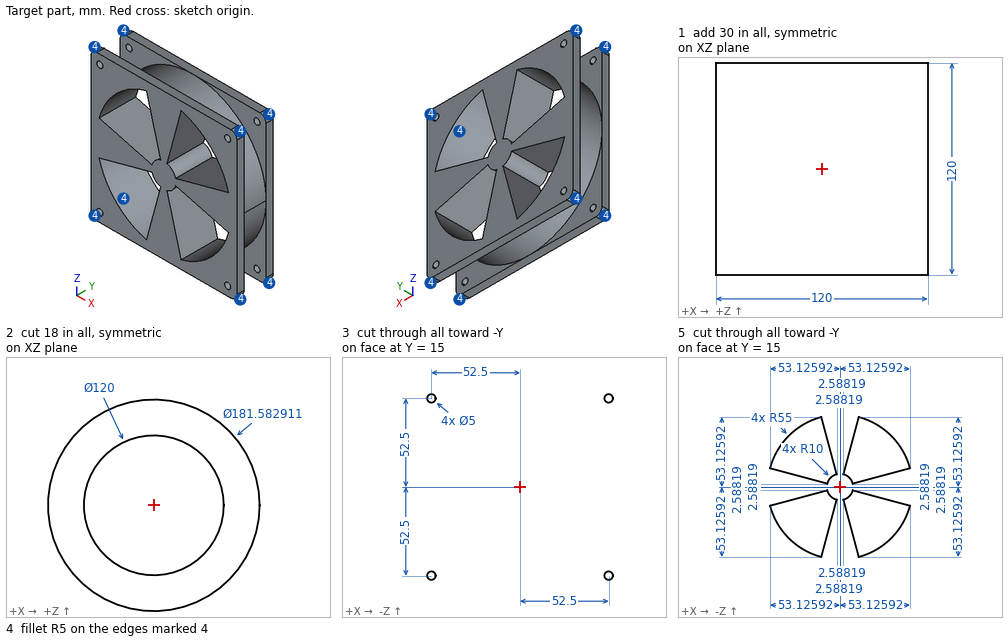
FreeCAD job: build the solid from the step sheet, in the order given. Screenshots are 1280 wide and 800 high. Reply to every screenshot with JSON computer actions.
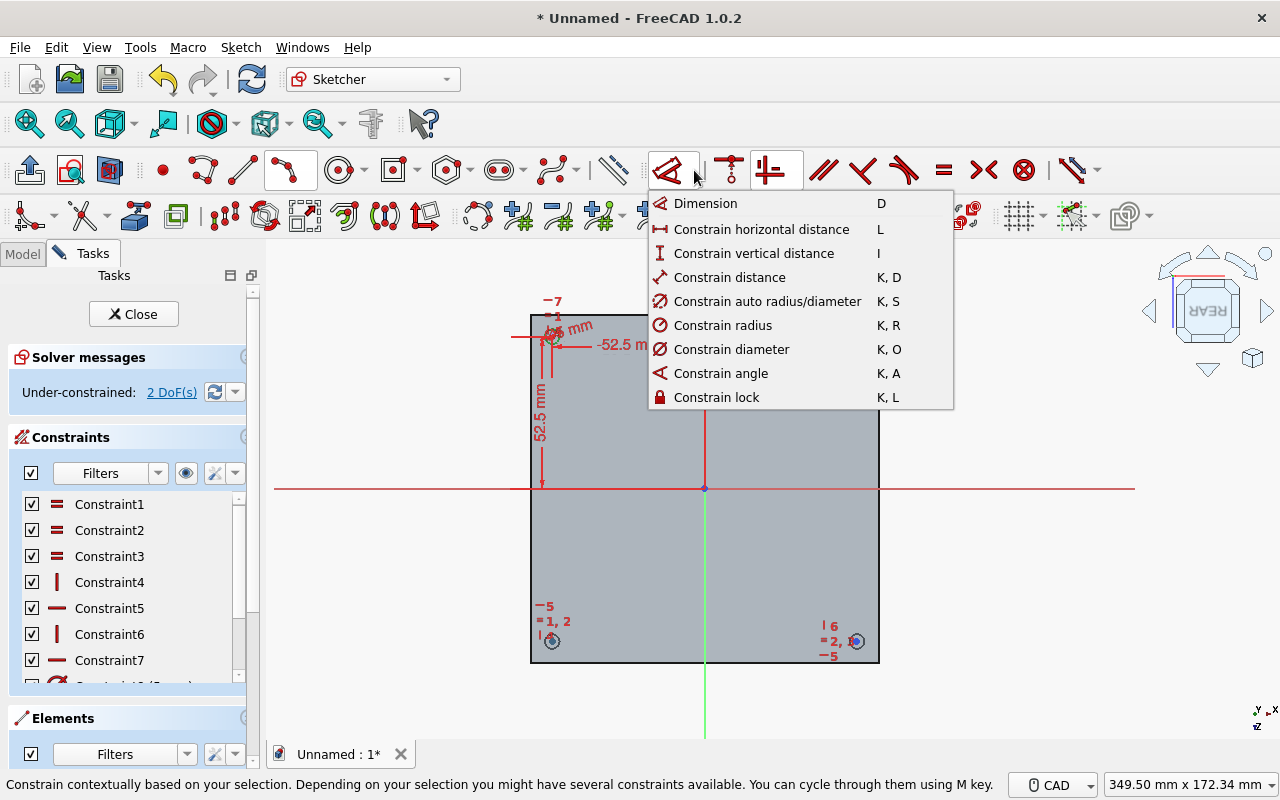
{"action": "left_click", "coordinate": [801, 253]}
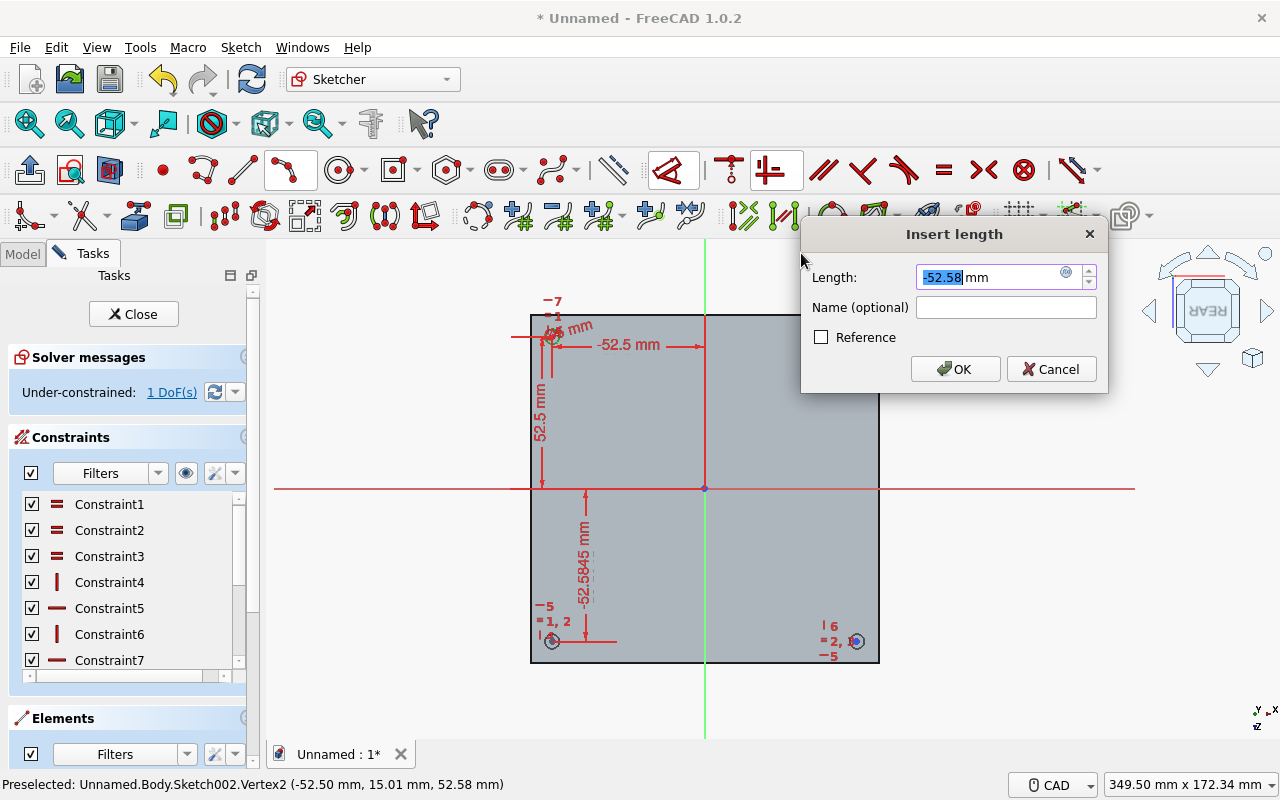
{"action": "type", "text": "-52.5"}
{"action": "key", "text": "Return"}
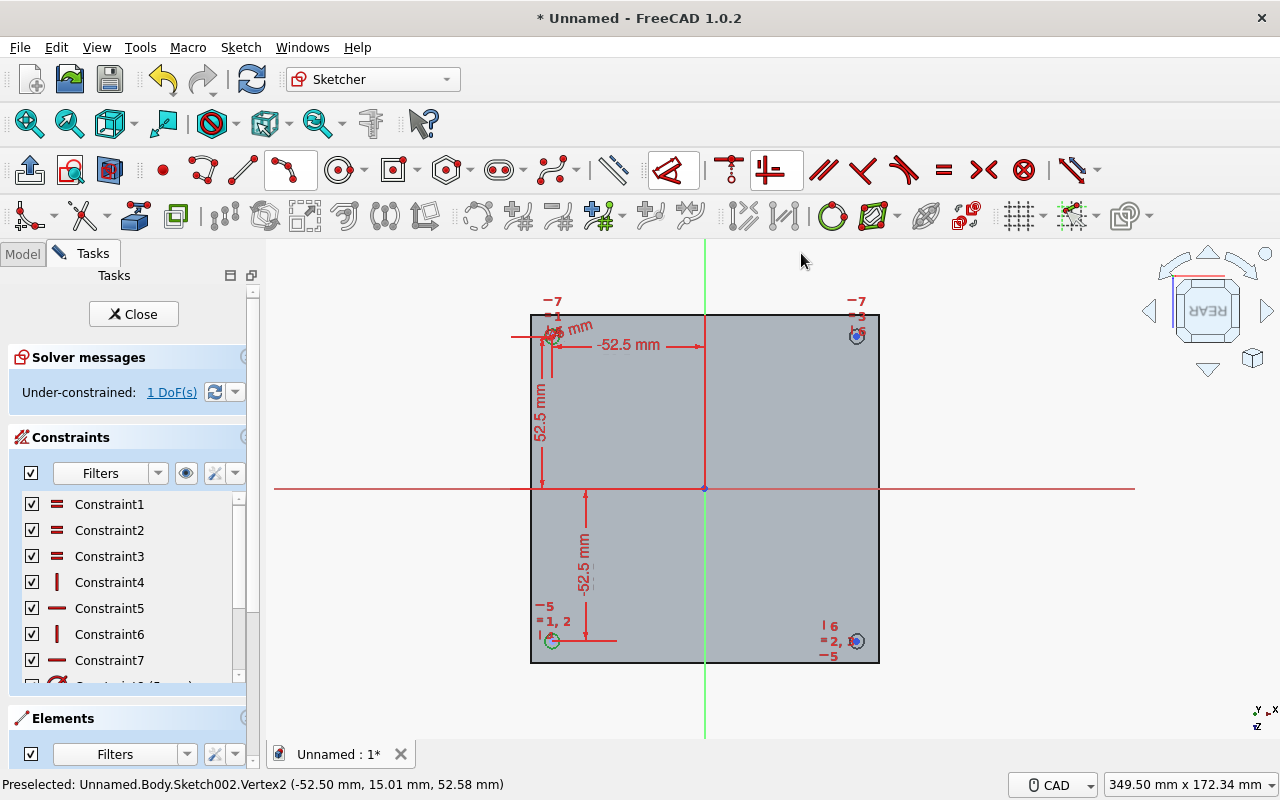
{"action": "left_click", "coordinate": [857, 641]}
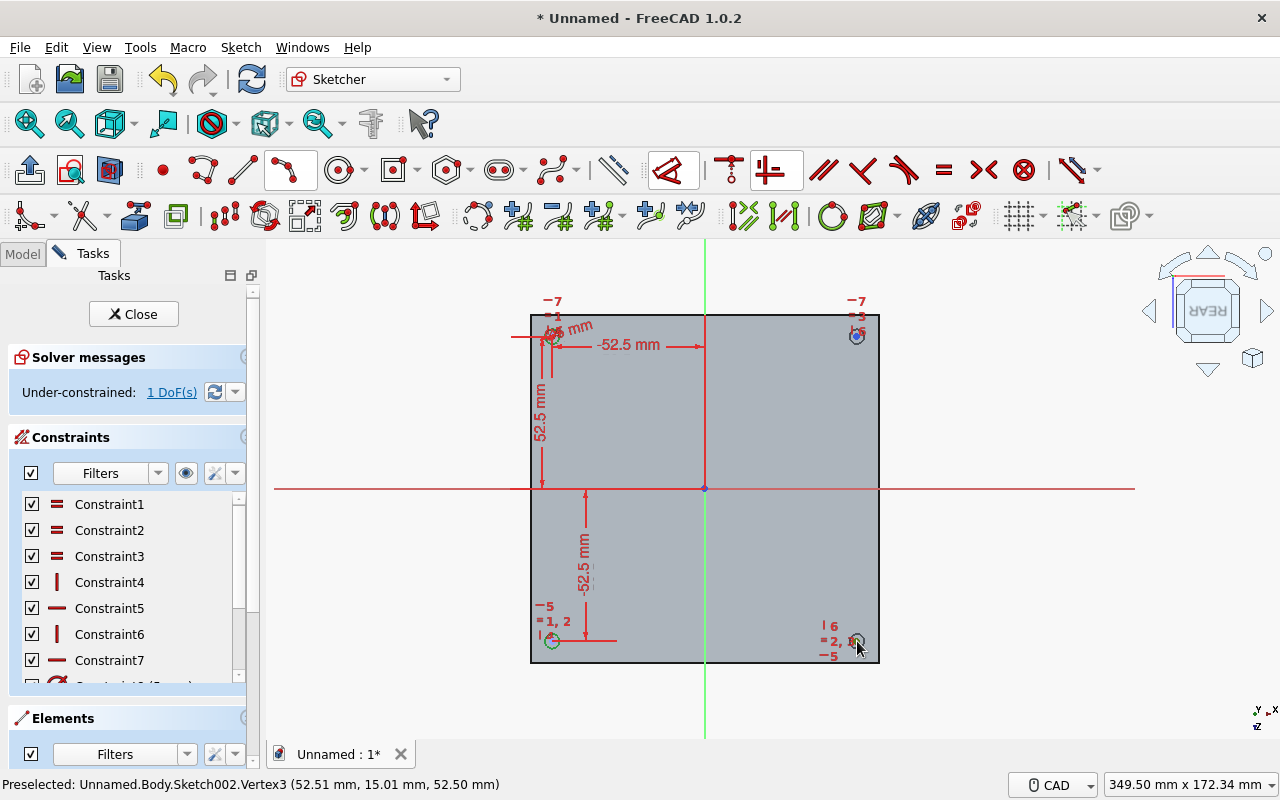
{"action": "key", "text": "l"}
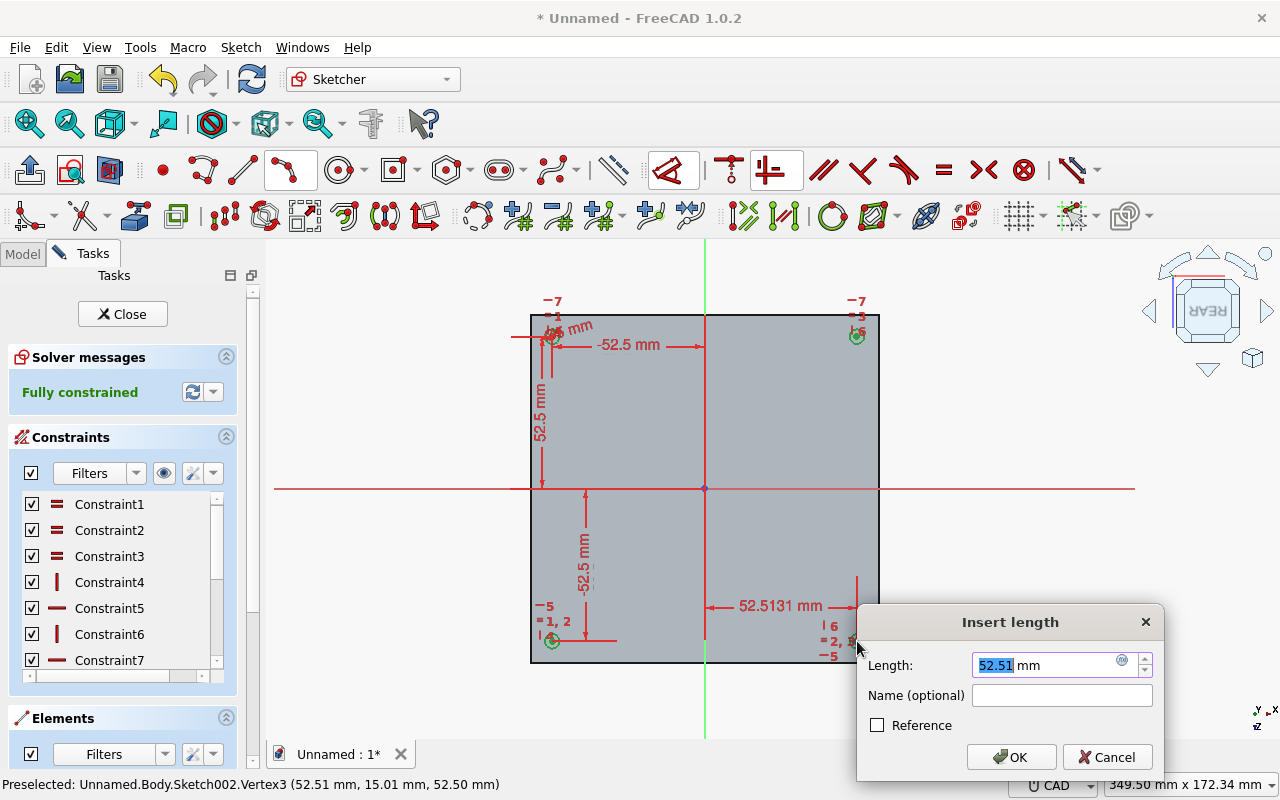
{"action": "type", "text": "52.5"}
{"action": "key", "text": "Return"}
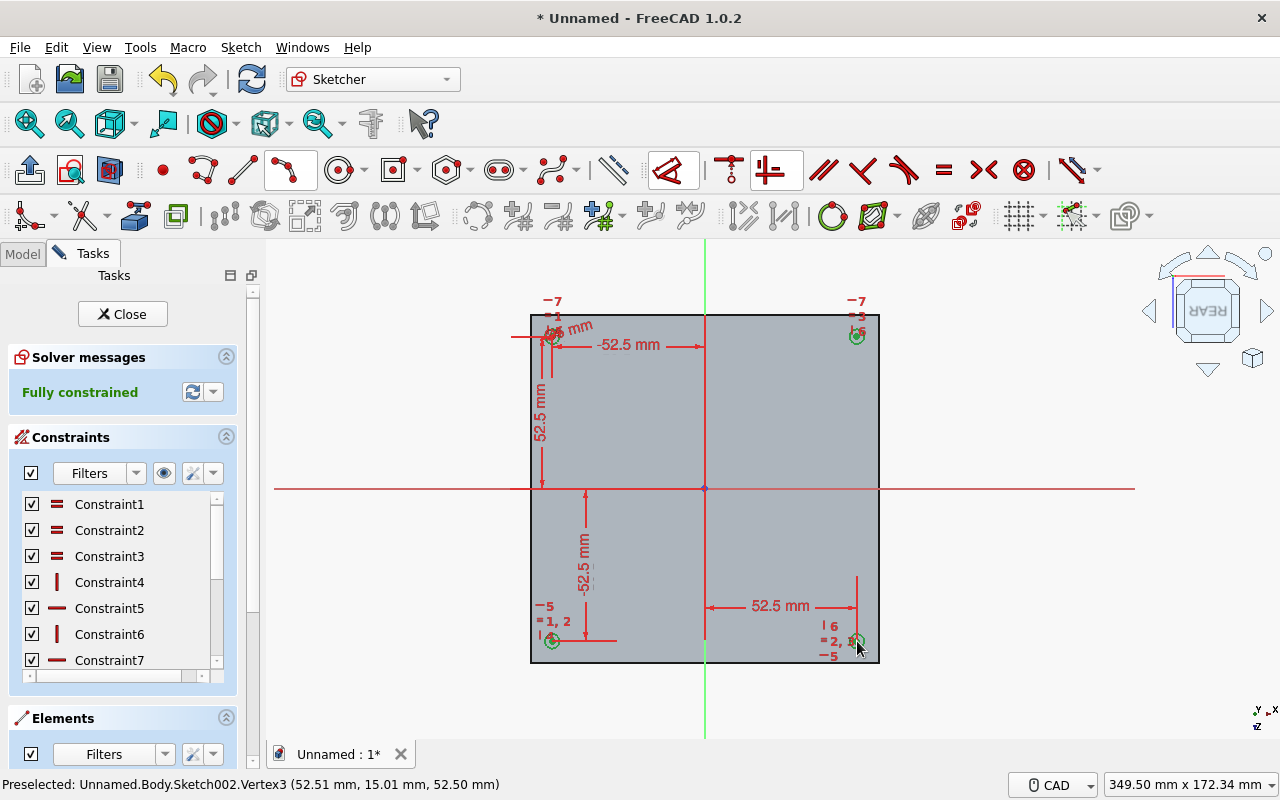
{"action": "left_click", "coordinate": [123, 314]}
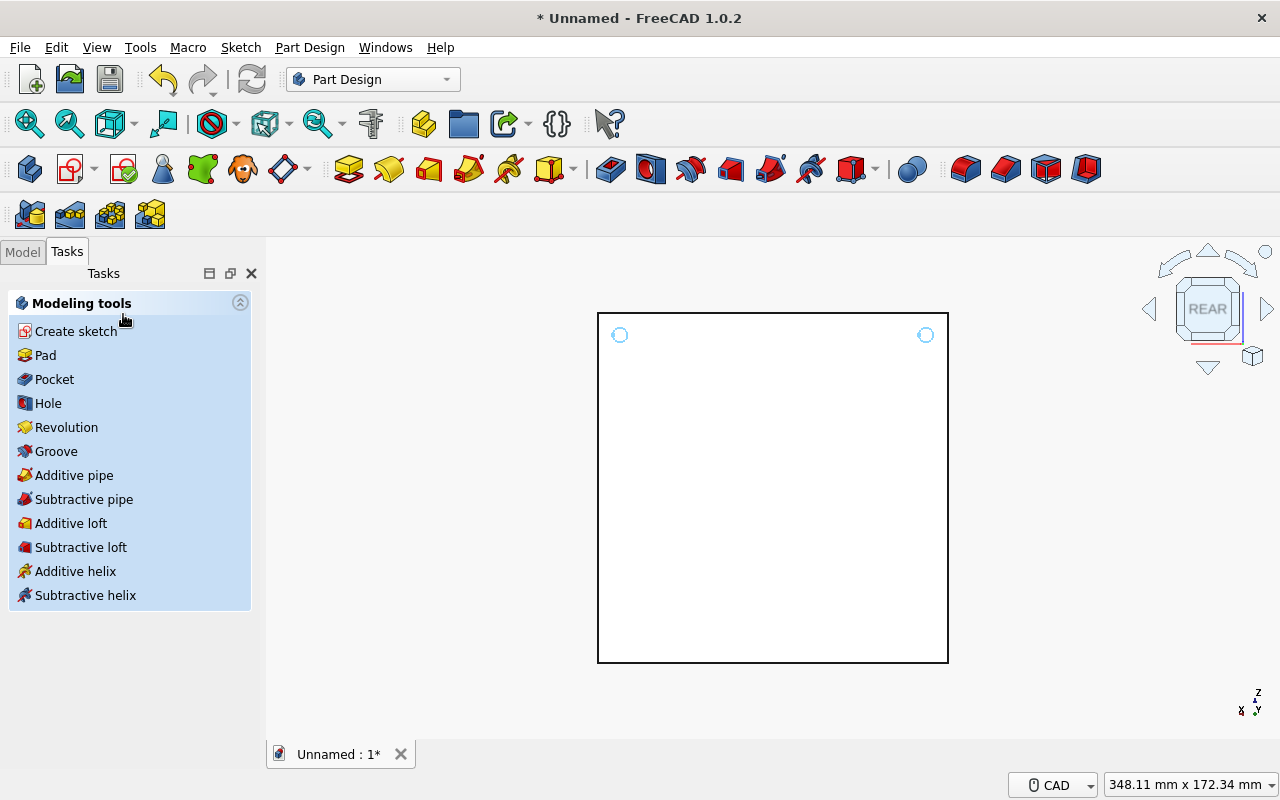
{"action": "left_click", "coordinate": [612, 170]}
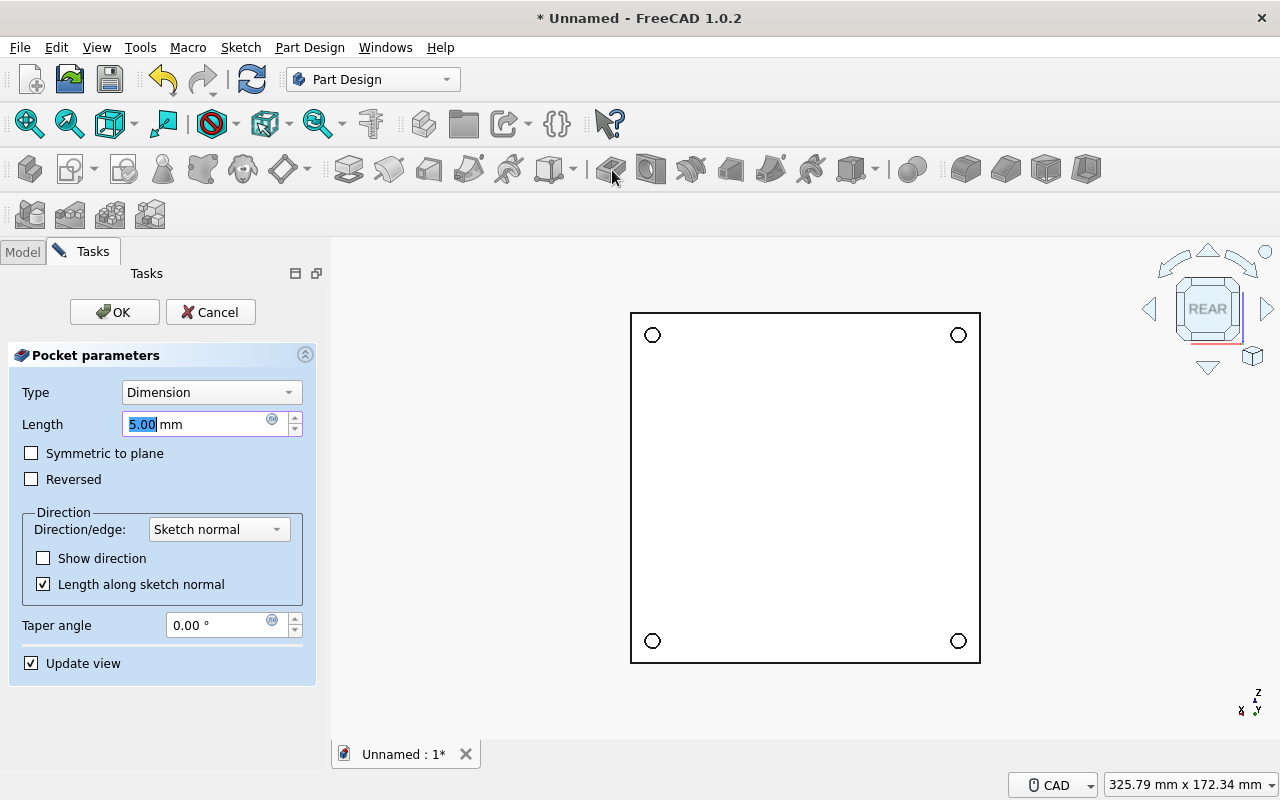
{"action": "left_click", "coordinate": [212, 392]}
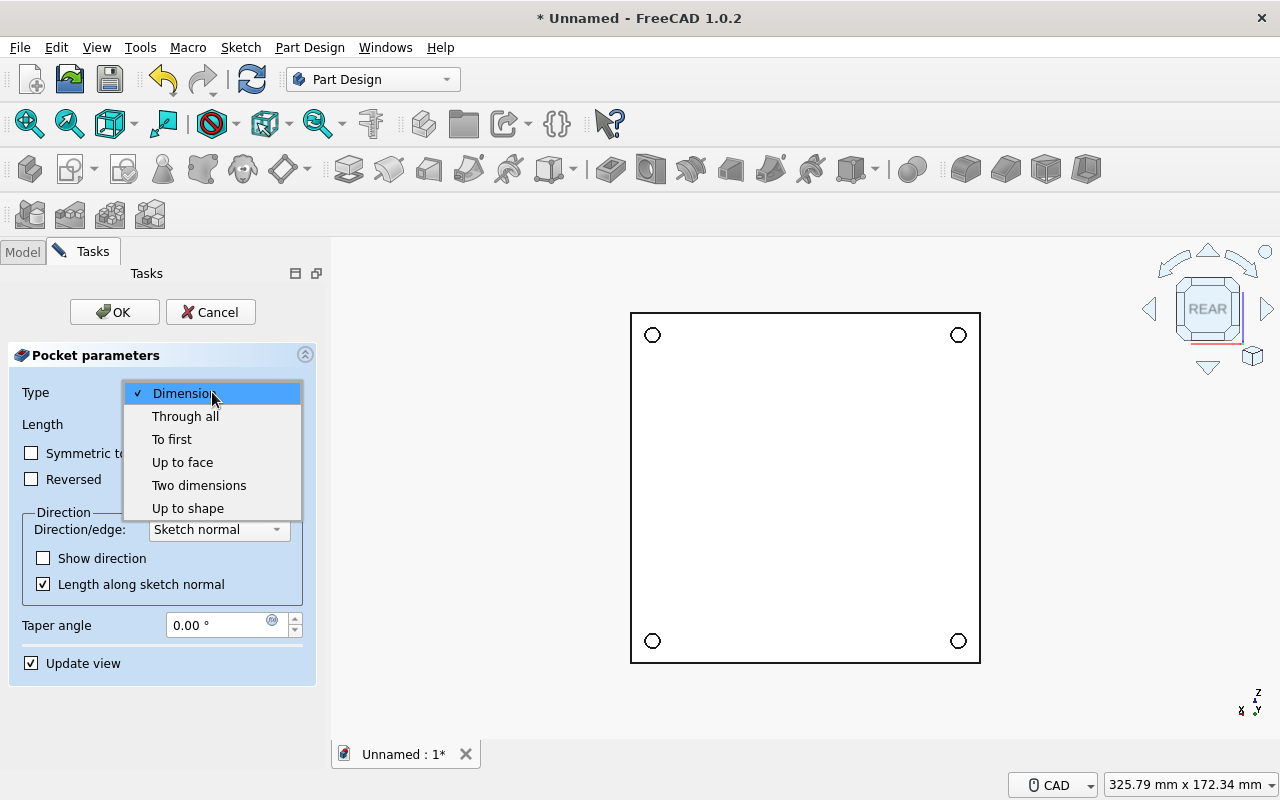
{"action": "left_click", "coordinate": [212, 416]}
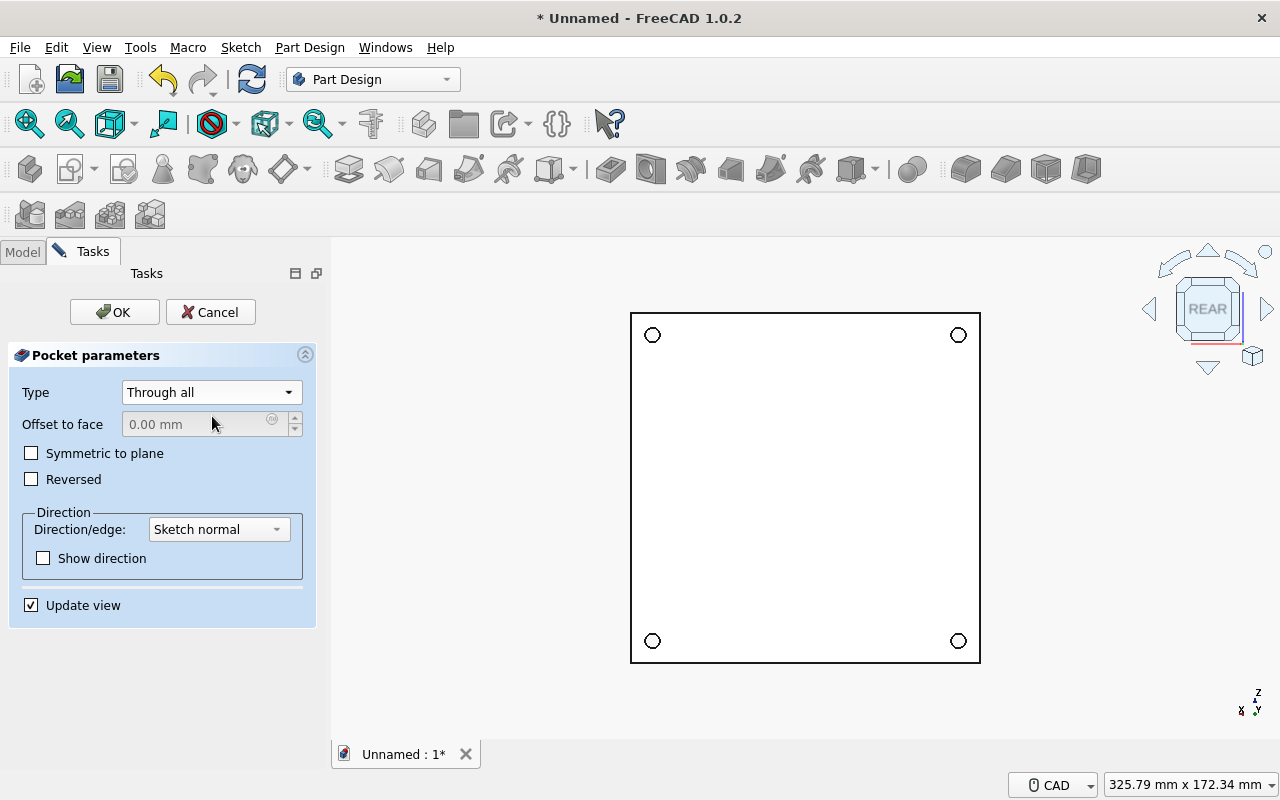
{"action": "left_click", "coordinate": [115, 312]}